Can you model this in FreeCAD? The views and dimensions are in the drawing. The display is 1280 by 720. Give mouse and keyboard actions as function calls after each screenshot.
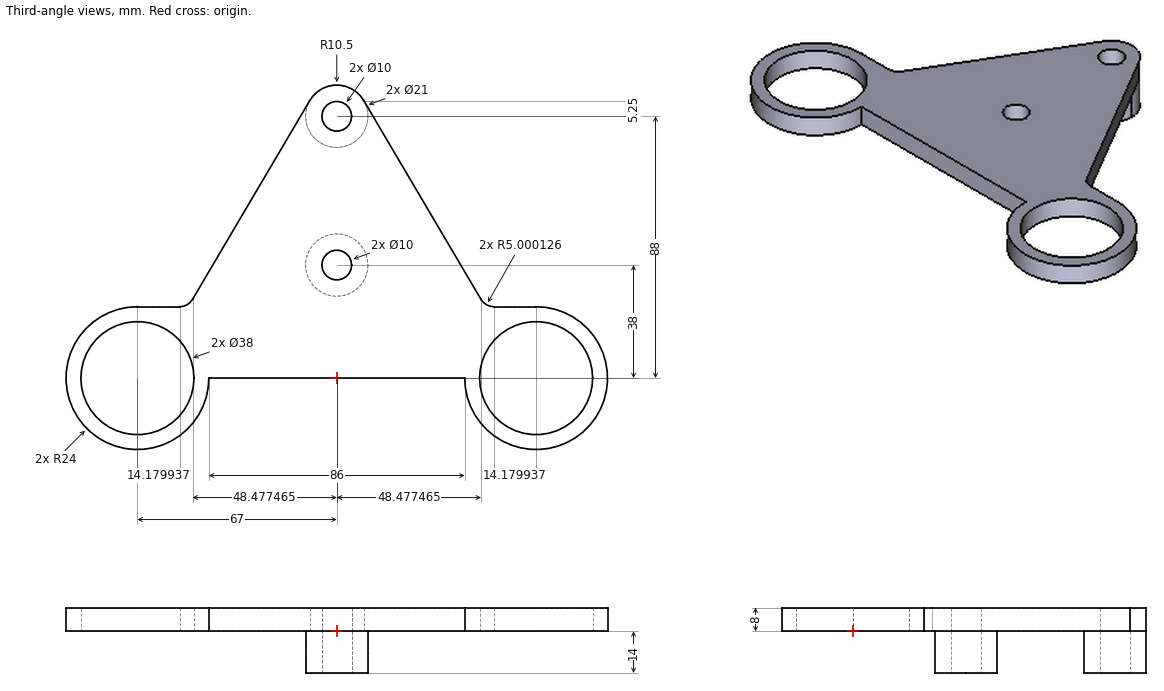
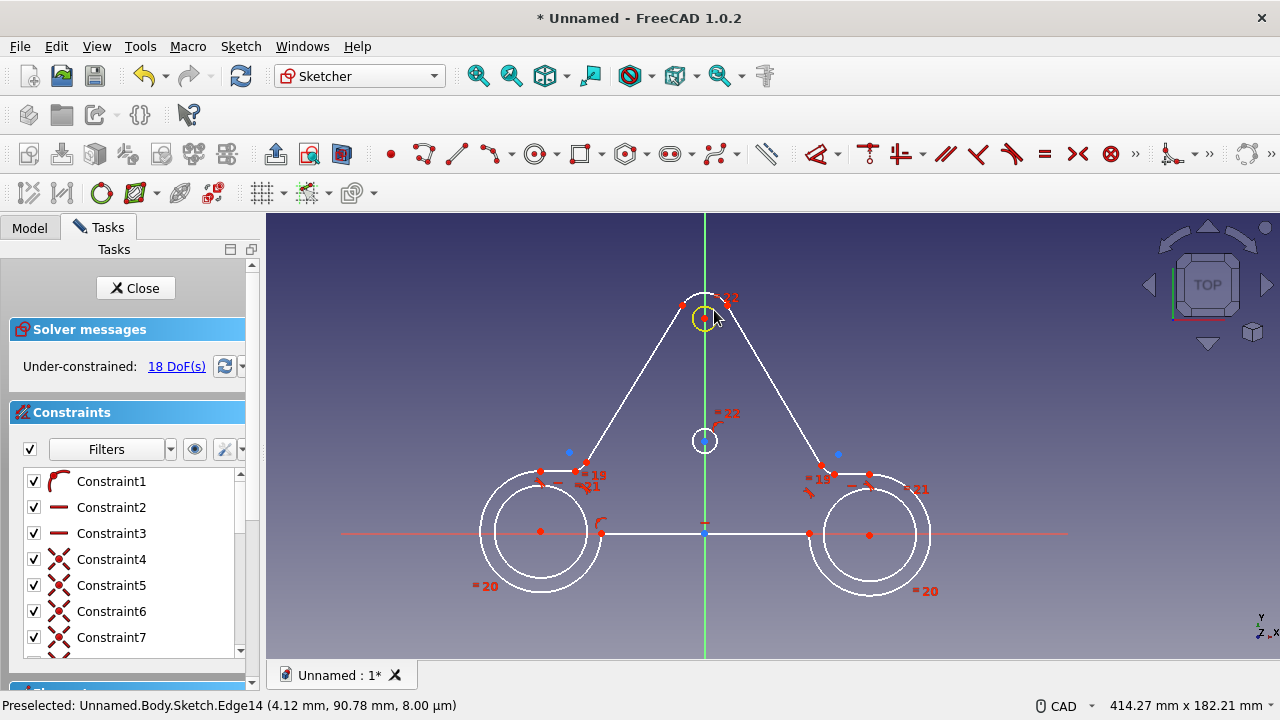
click(870, 535)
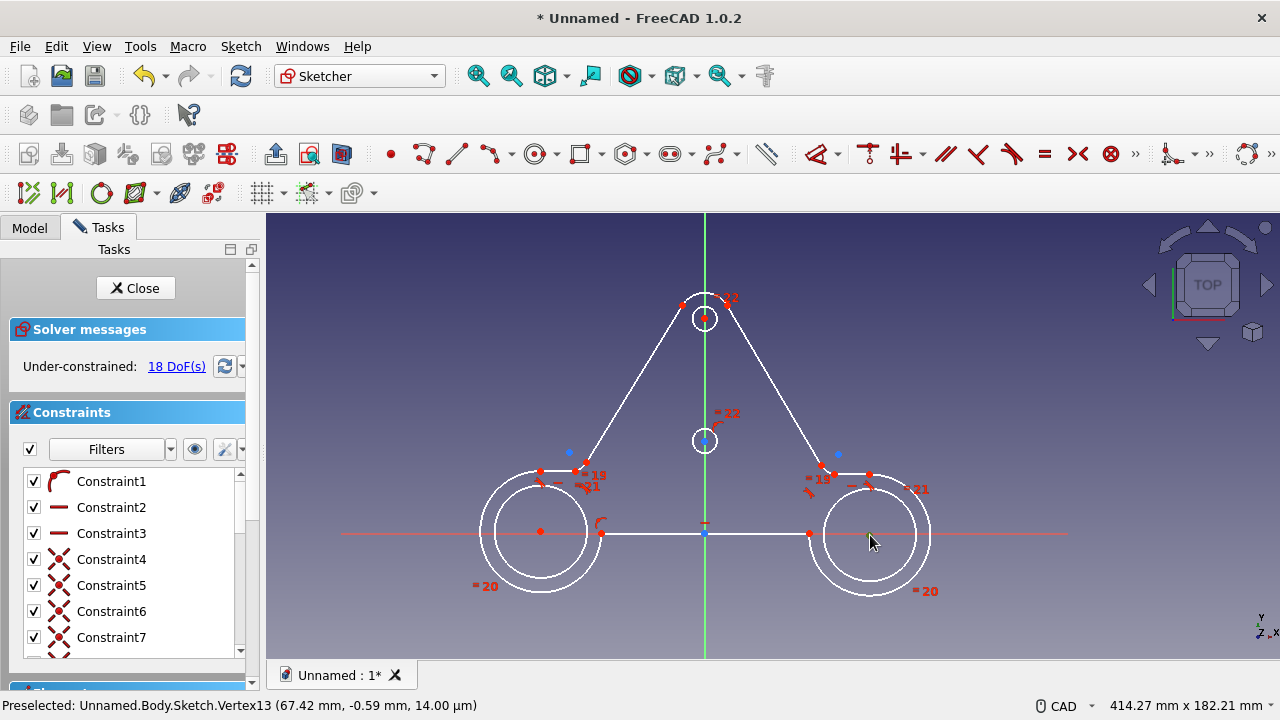
click(353, 534)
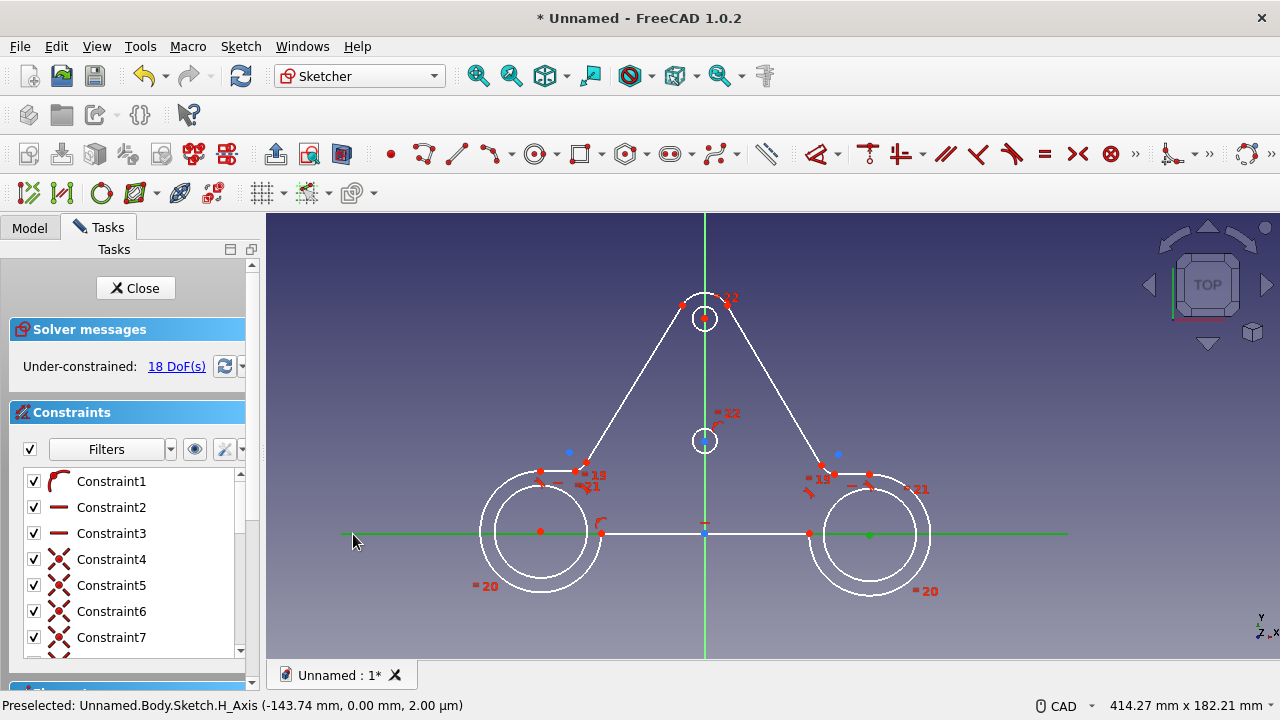
click(868, 154)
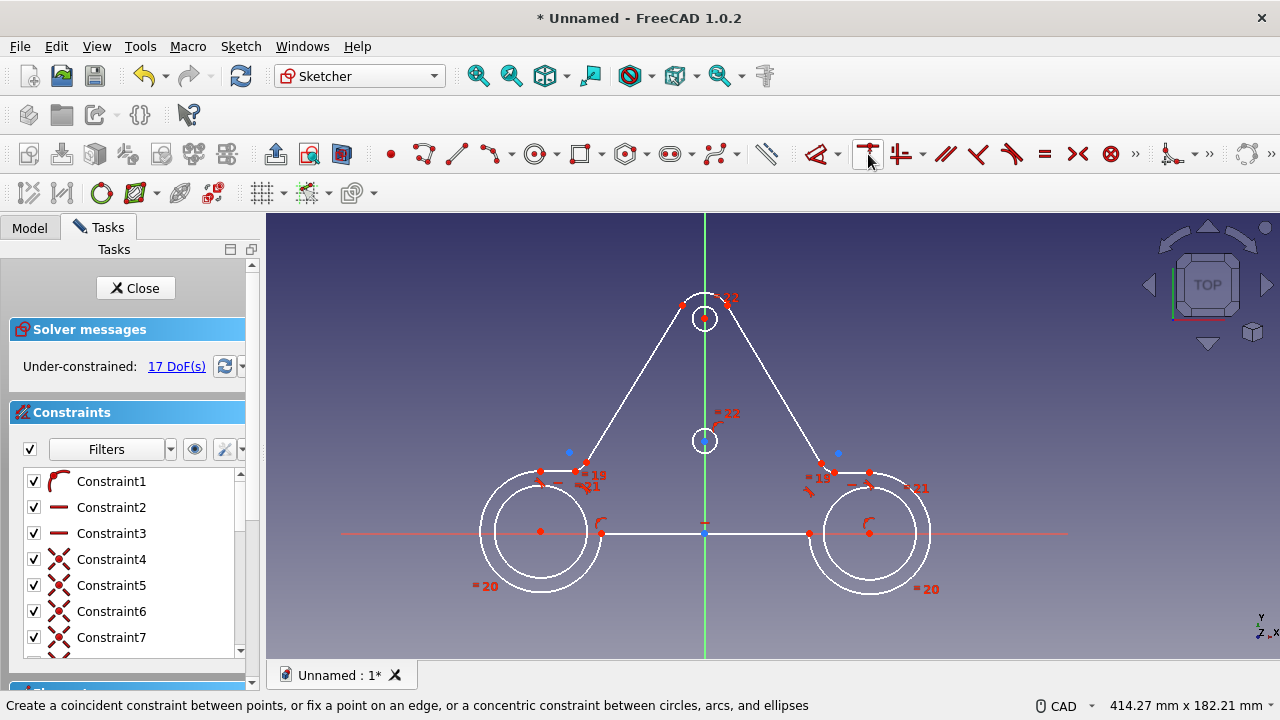
click(705, 319)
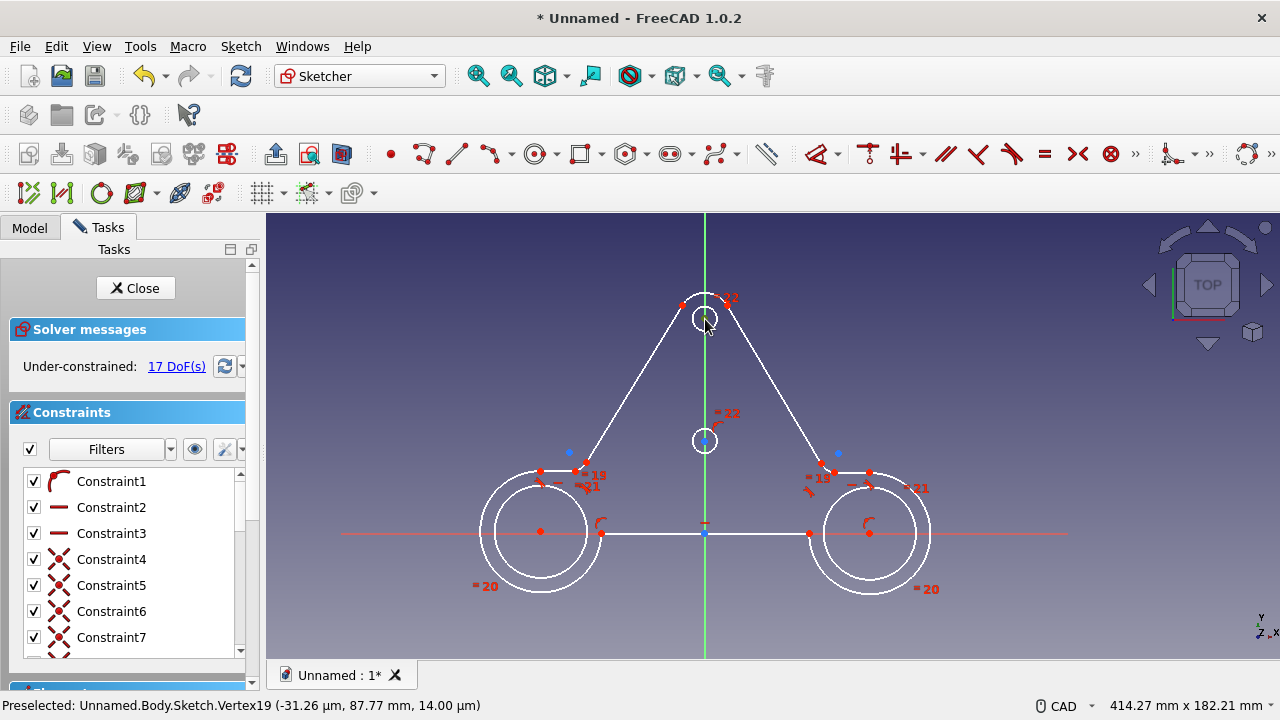
click(705, 603)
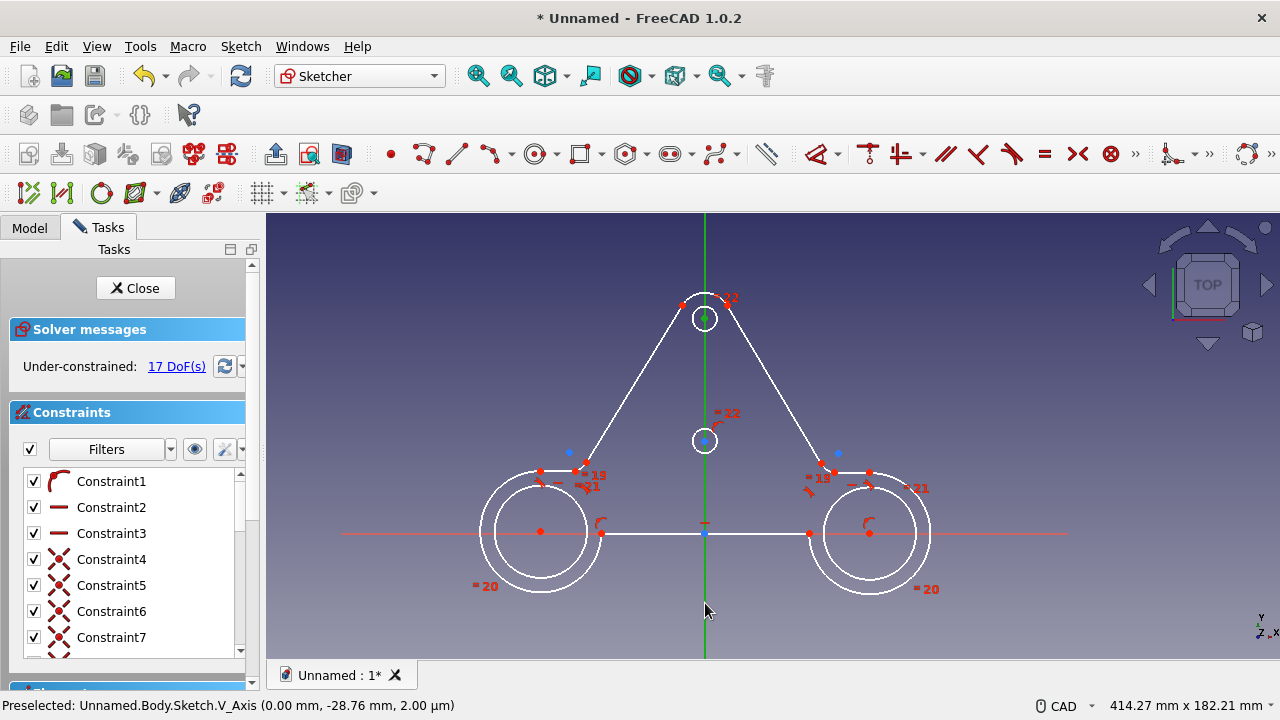
click(868, 154)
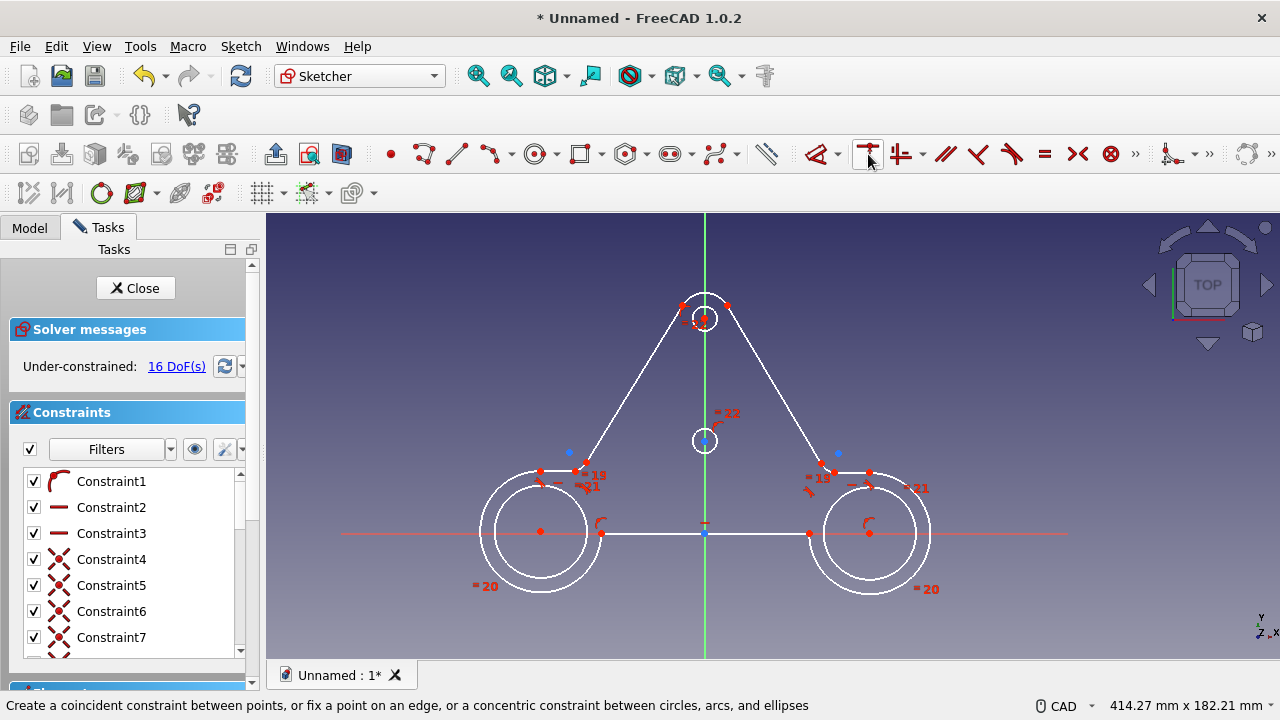
click(541, 532)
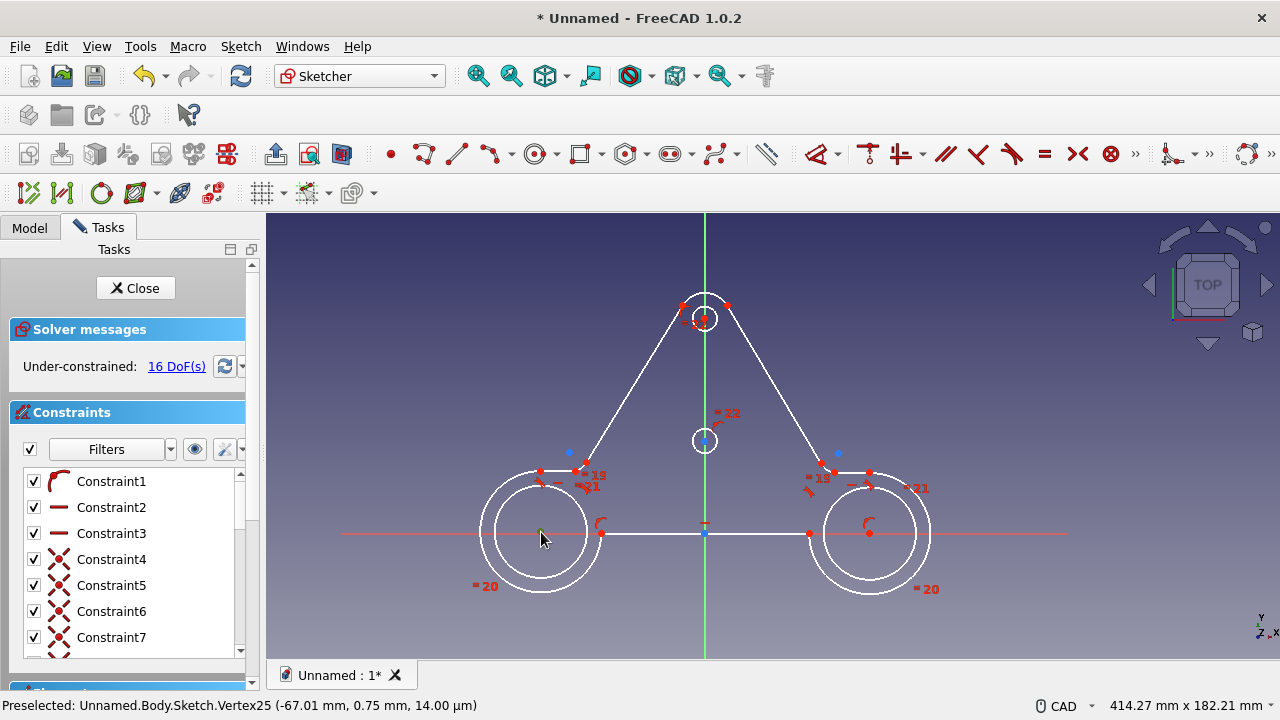
click(353, 534)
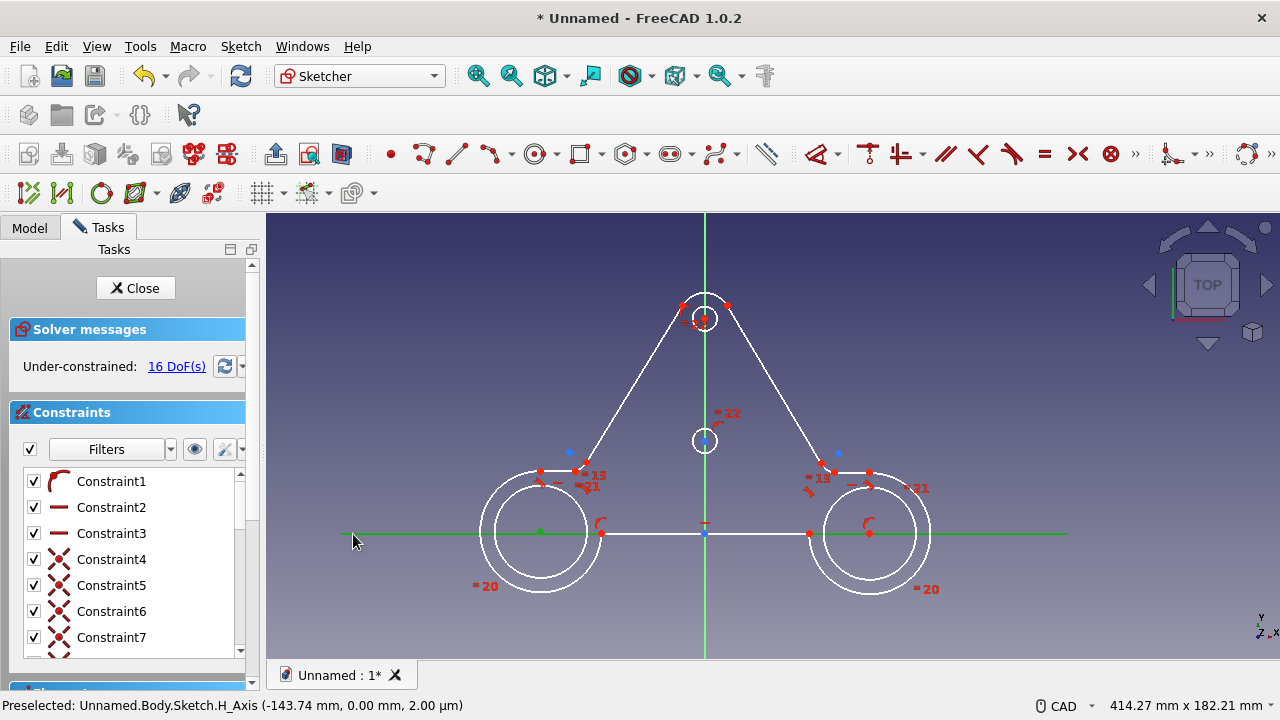
key(c)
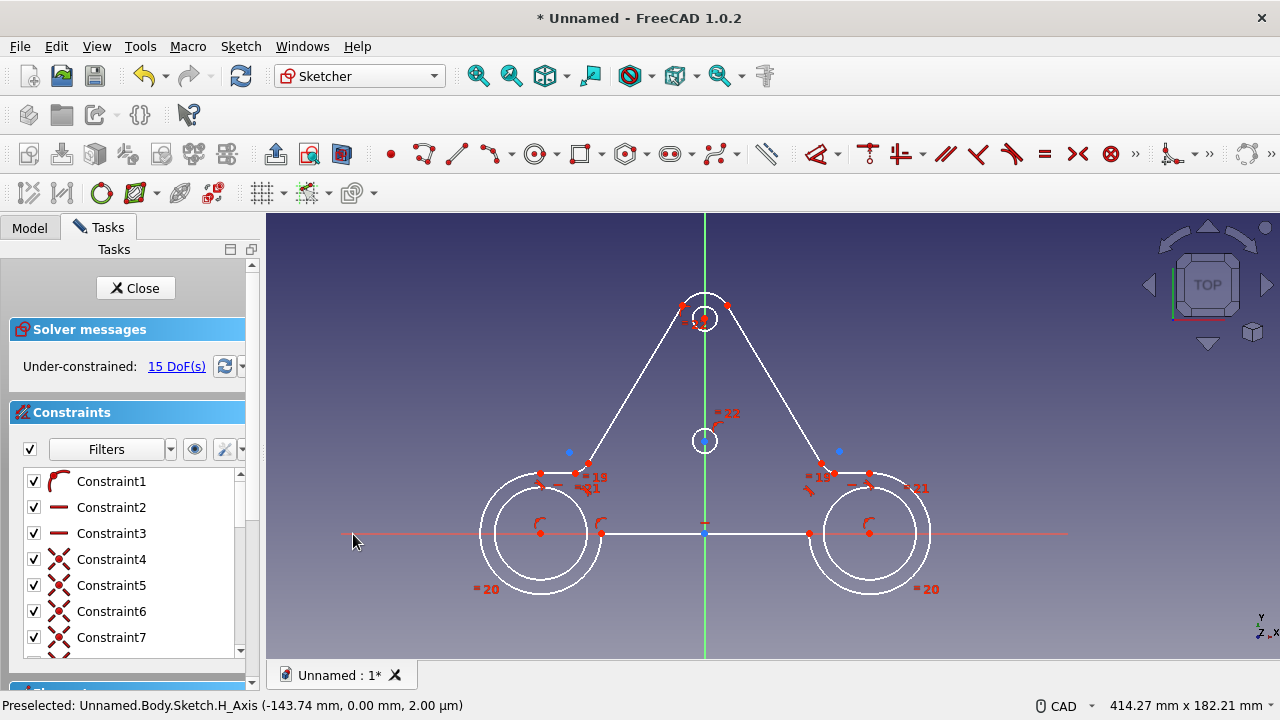
click(816, 154)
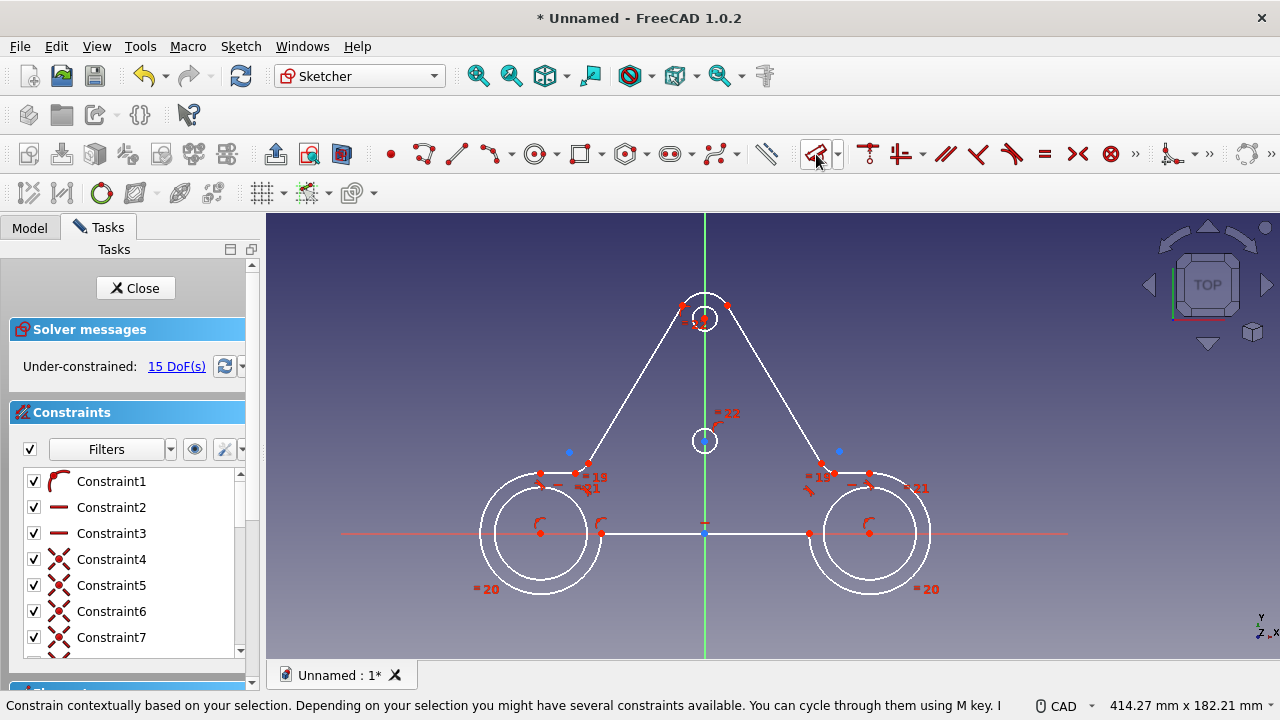
click(860, 593)
click(855, 625)